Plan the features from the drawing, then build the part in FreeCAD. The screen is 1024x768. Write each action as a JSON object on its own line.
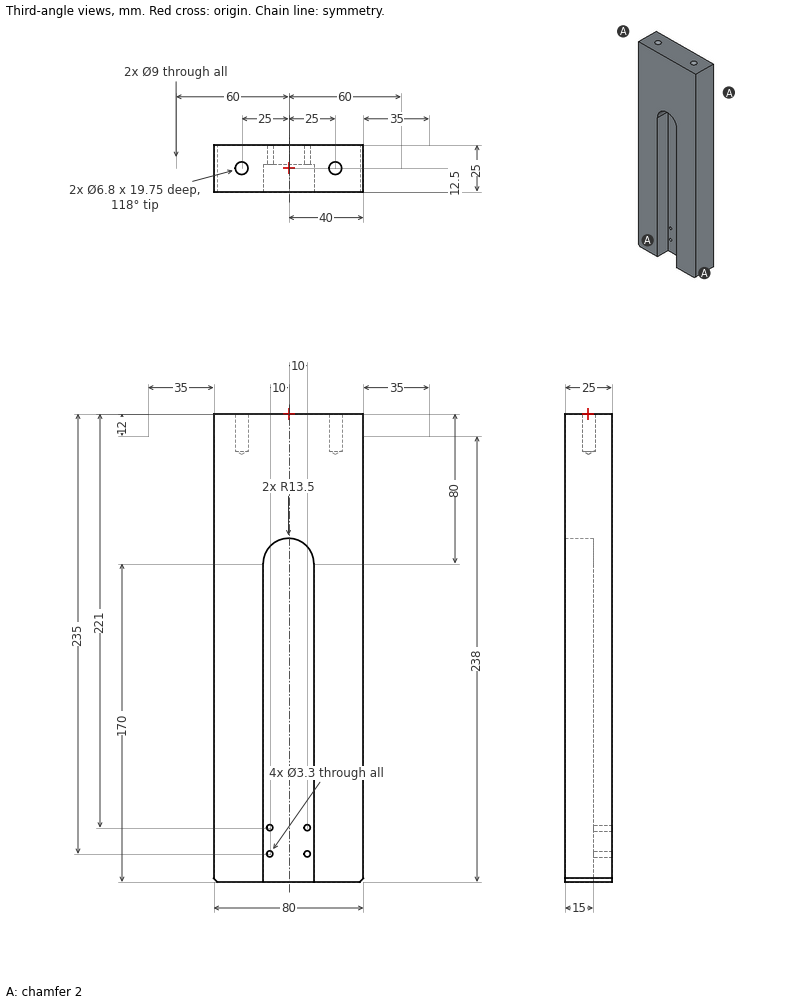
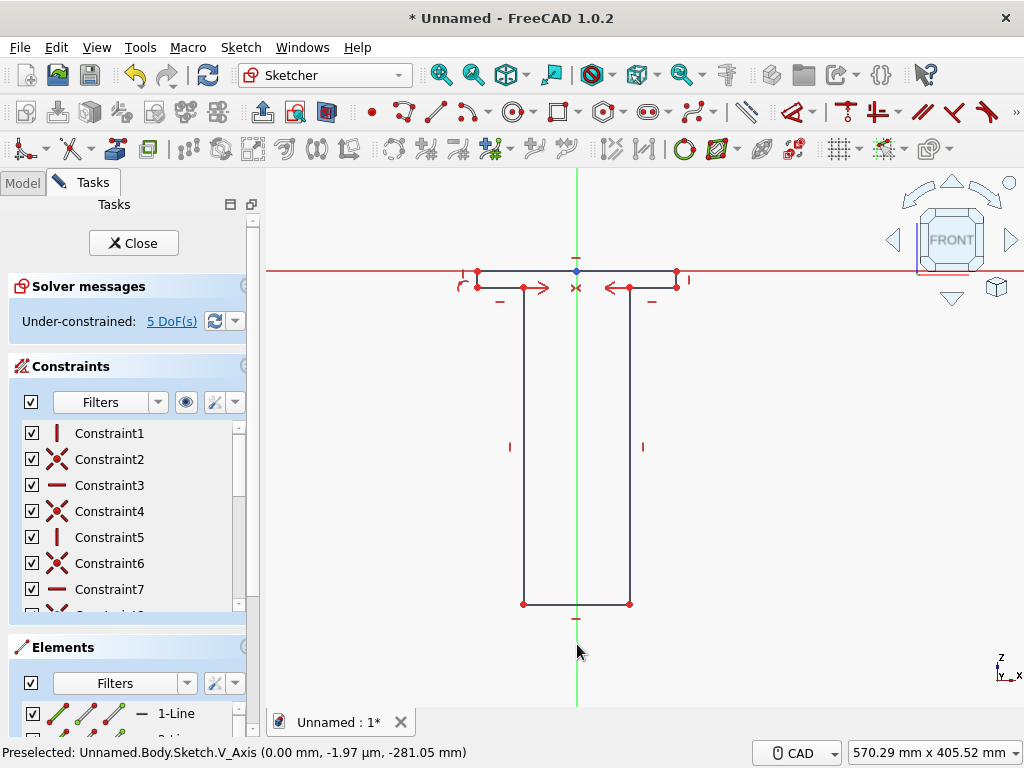
{"action": "key", "text": "d"}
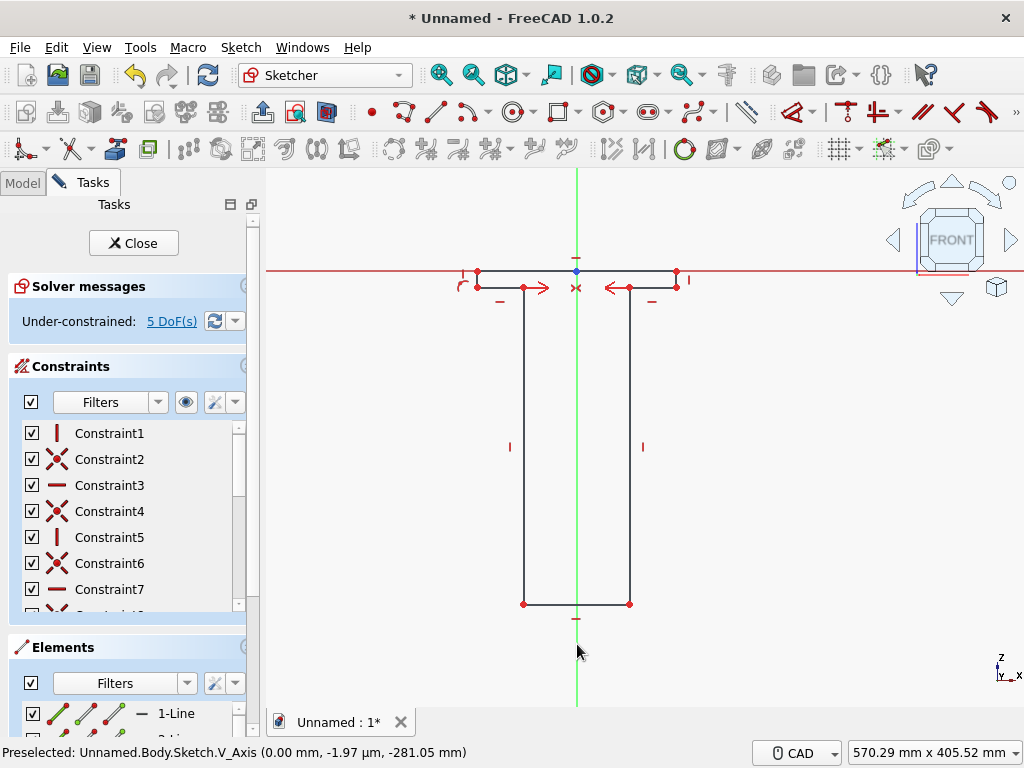
{"action": "left_click", "coordinate": [598, 605]}
{"action": "left_click", "coordinate": [552, 639]}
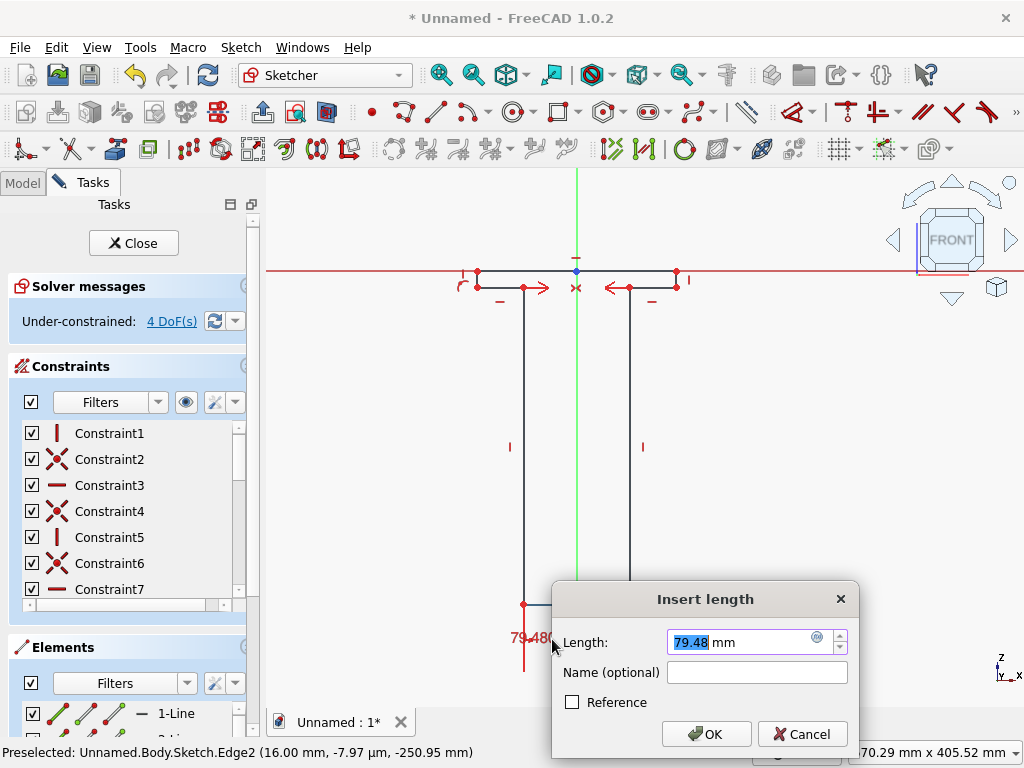
{"action": "type", "text": "80"}
{"action": "key", "text": "Return"}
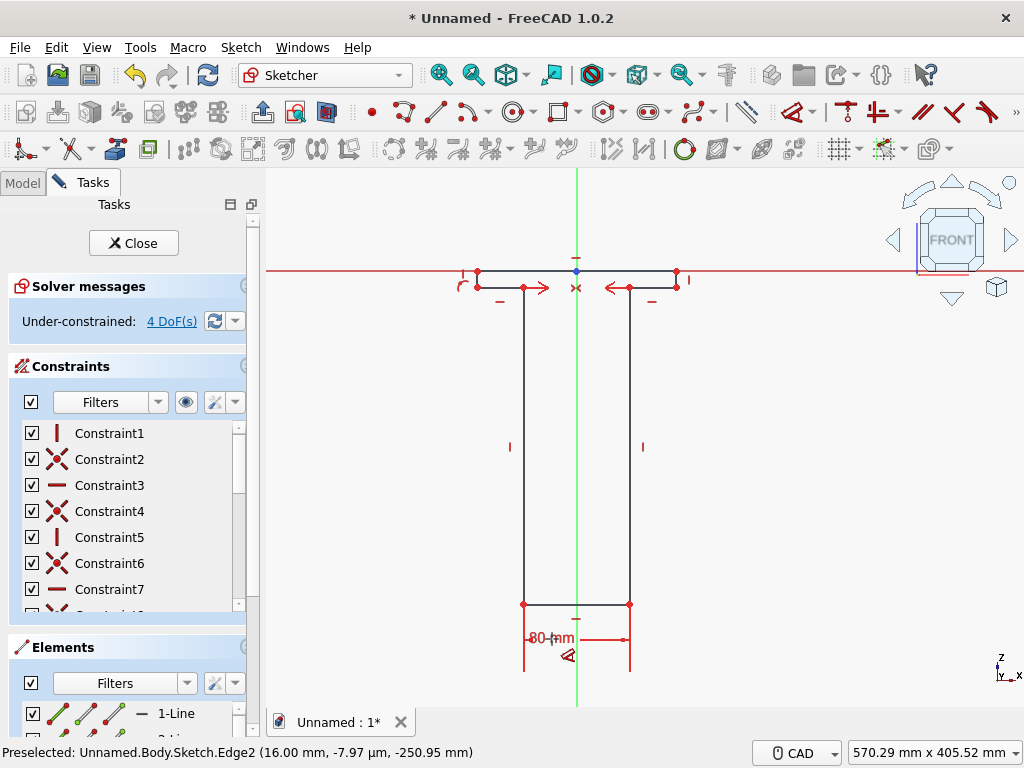
{"action": "left_click", "coordinate": [510, 288]}
{"action": "left_click", "coordinate": [500, 254]}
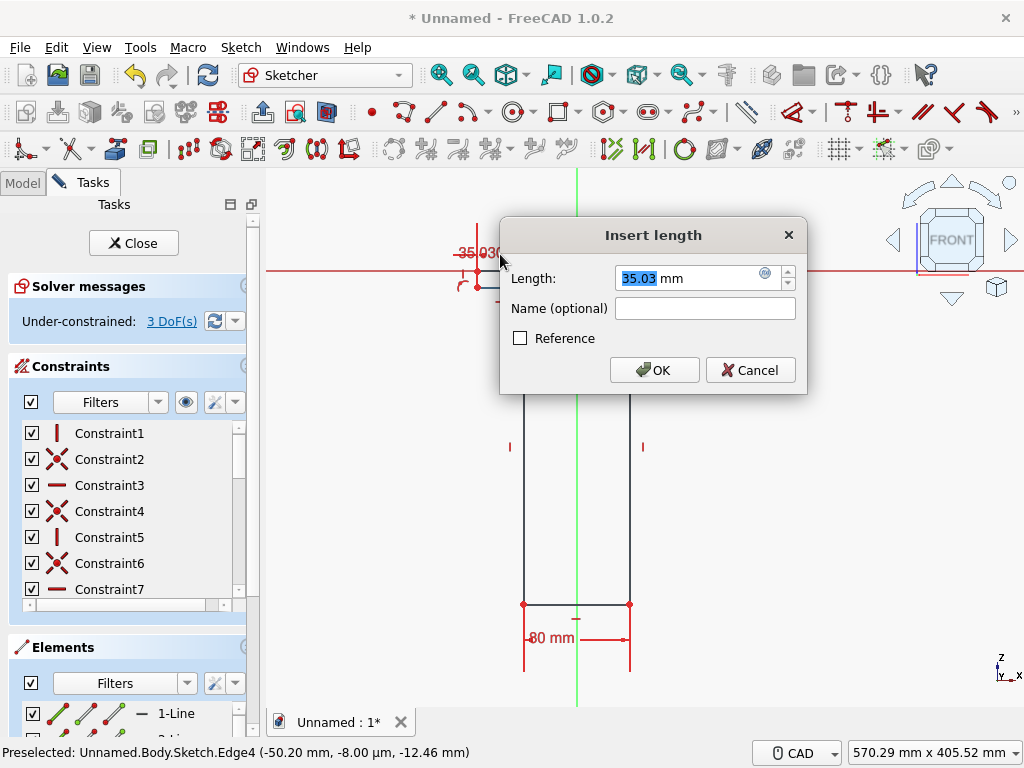
{"action": "type", "text": "35"}
{"action": "key", "text": "Return"}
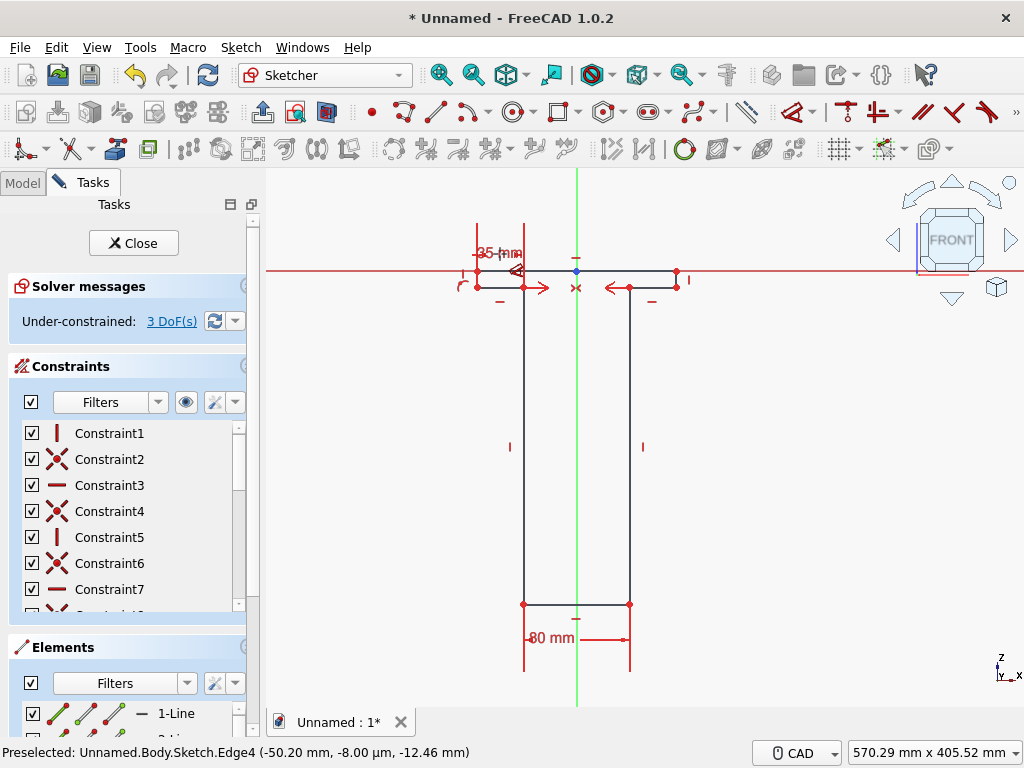
{"action": "scroll", "coordinate": [477, 280], "scroll_direction": "up", "scroll_amount": 5}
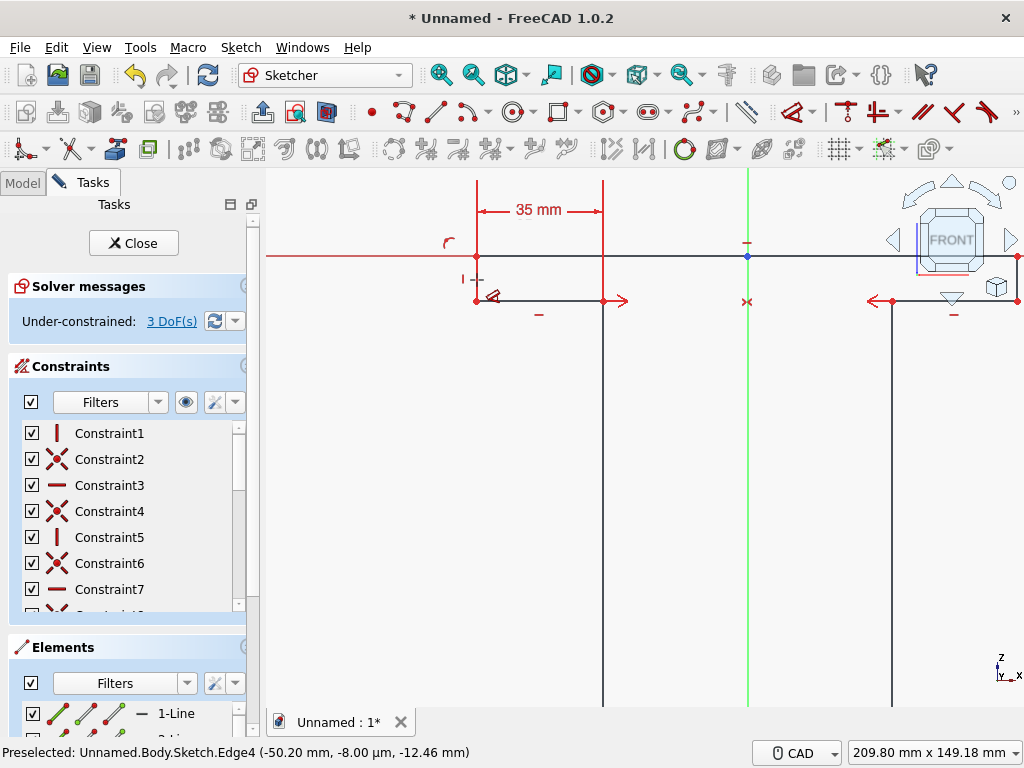
{"action": "left_click", "coordinate": [477, 279]}
{"action": "left_click", "coordinate": [443, 279]}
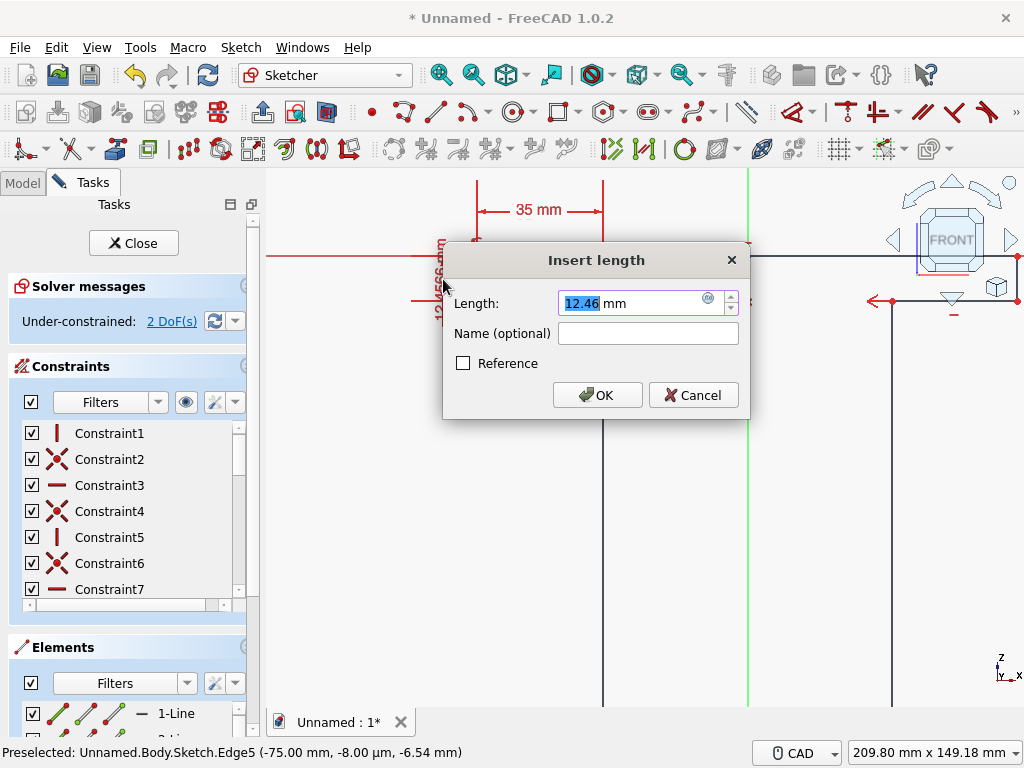
{"action": "type", "text": "12"}
{"action": "key", "text": "Return"}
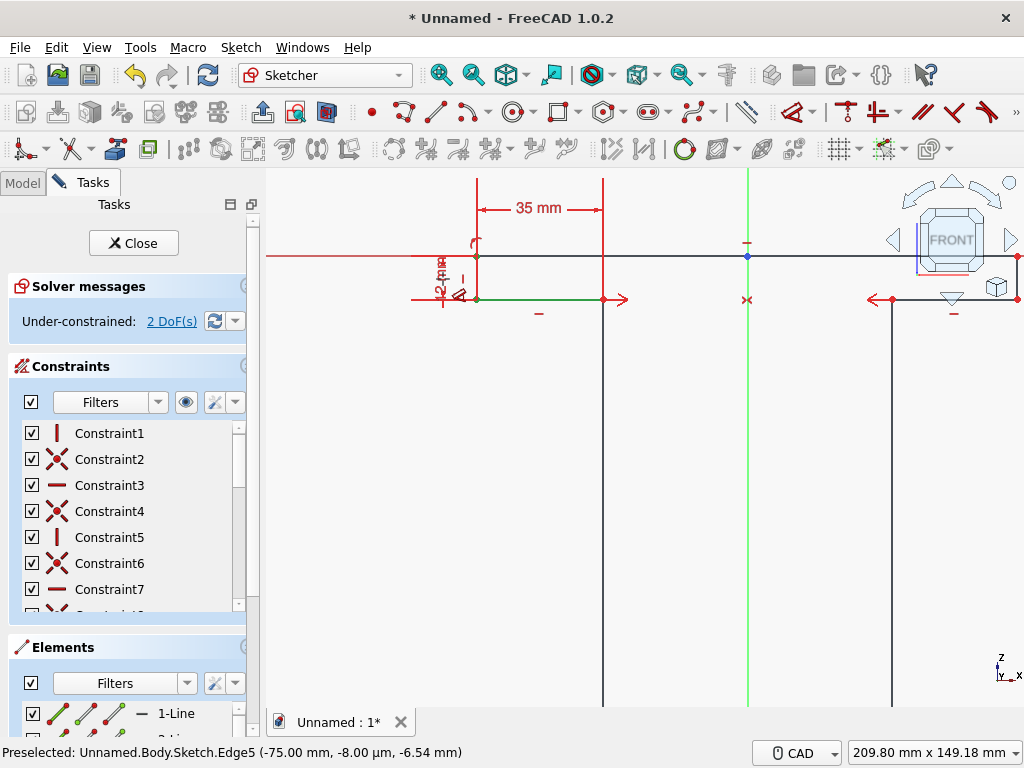
{"action": "scroll", "coordinate": [477, 280], "scroll_direction": "down", "scroll_amount": 5}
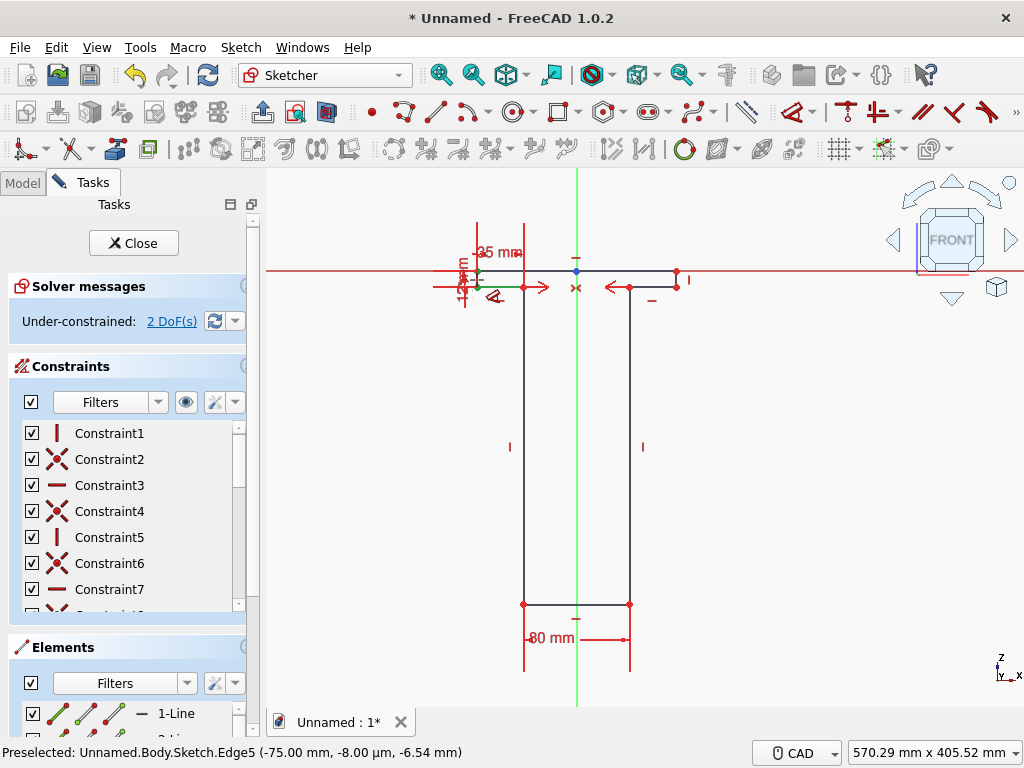
{"action": "left_click", "coordinate": [662, 287]}
{"action": "left_click", "coordinate": [653, 253]}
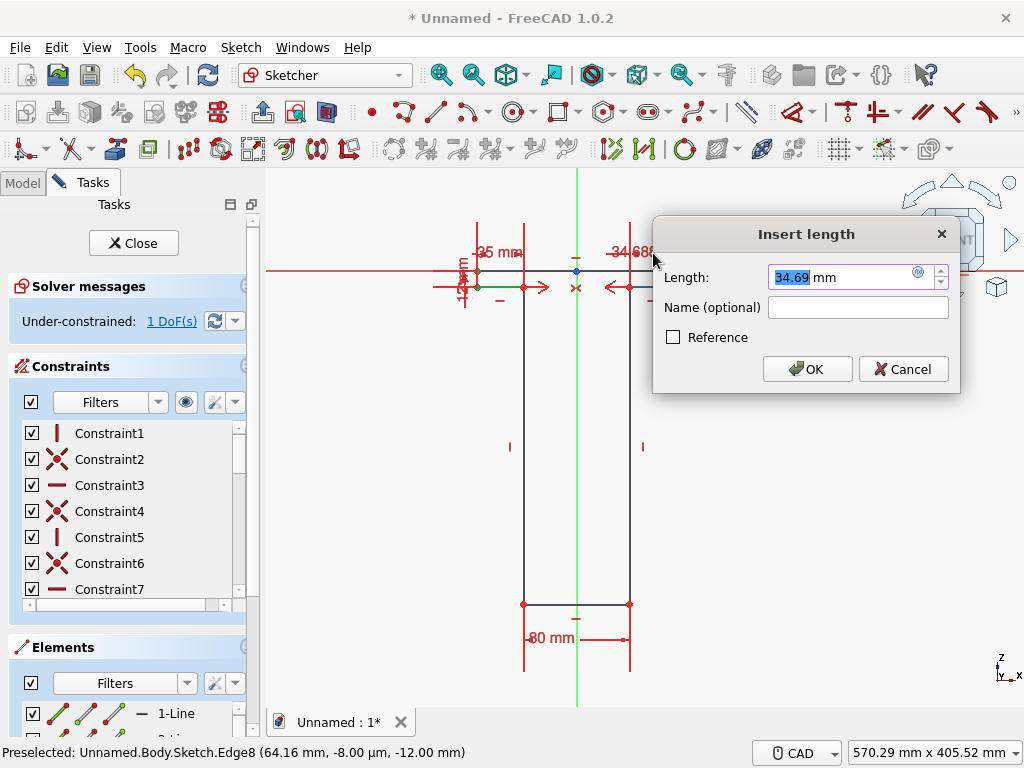
{"action": "type", "text": "35"}
{"action": "key", "text": "Return"}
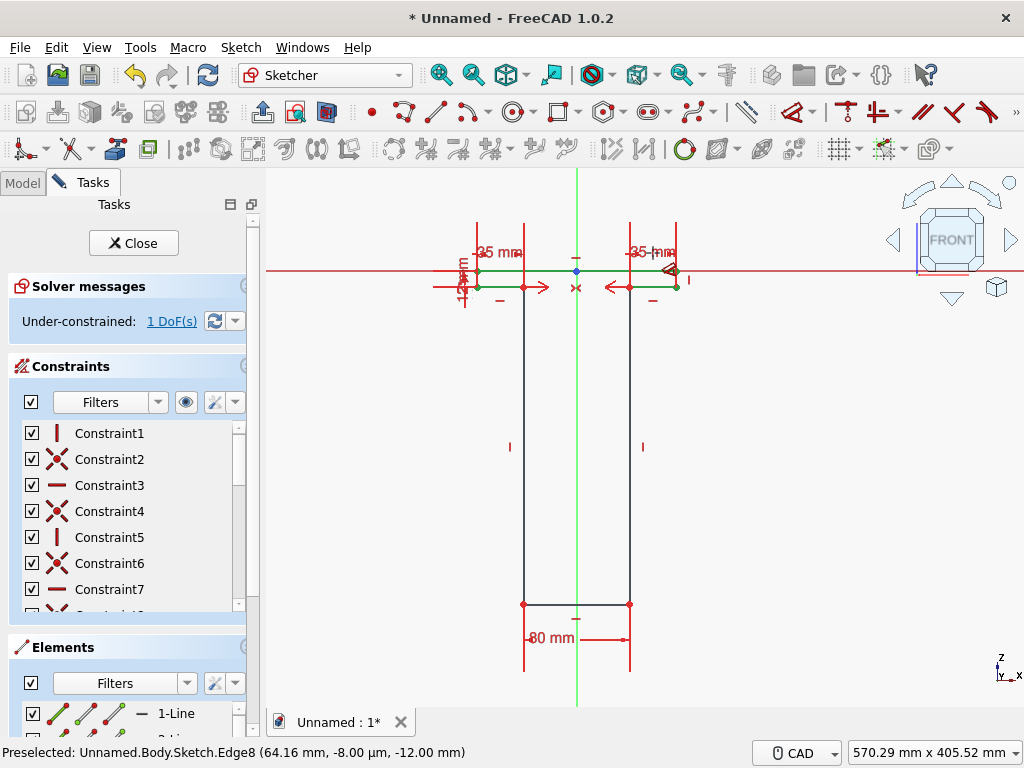
{"action": "left_click", "coordinate": [630, 383]}
{"action": "left_click", "coordinate": [664, 446]}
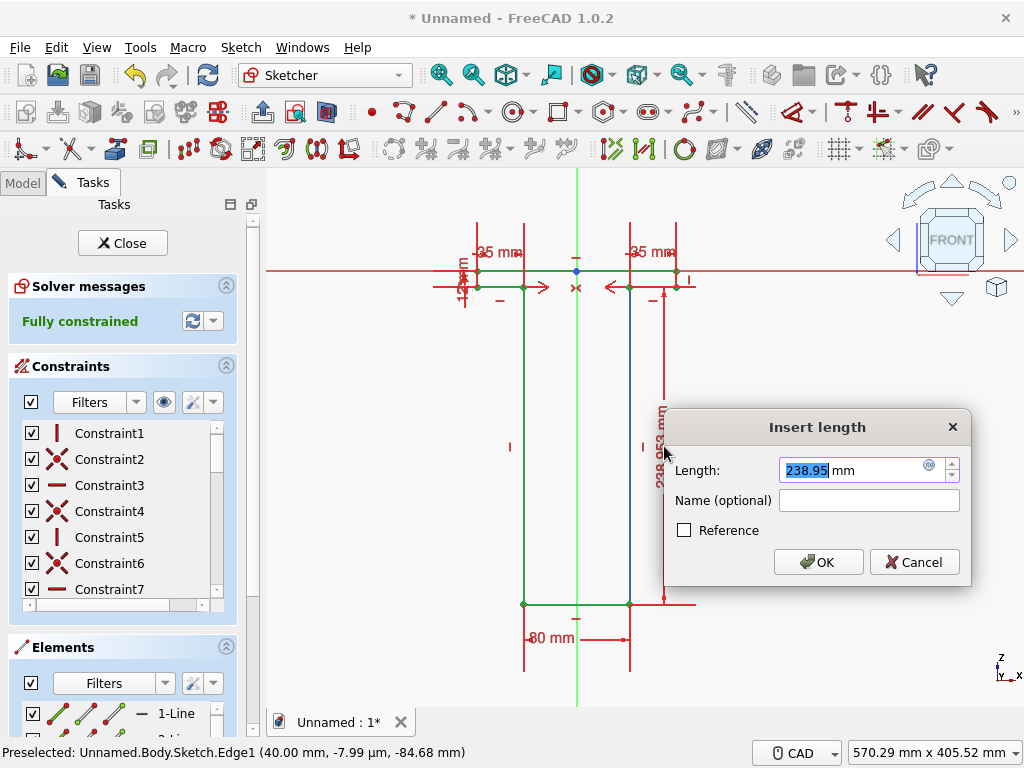
{"action": "type", "text": "238"}
{"action": "key", "text": "Return"}
{"action": "key", "text": "Escape"}